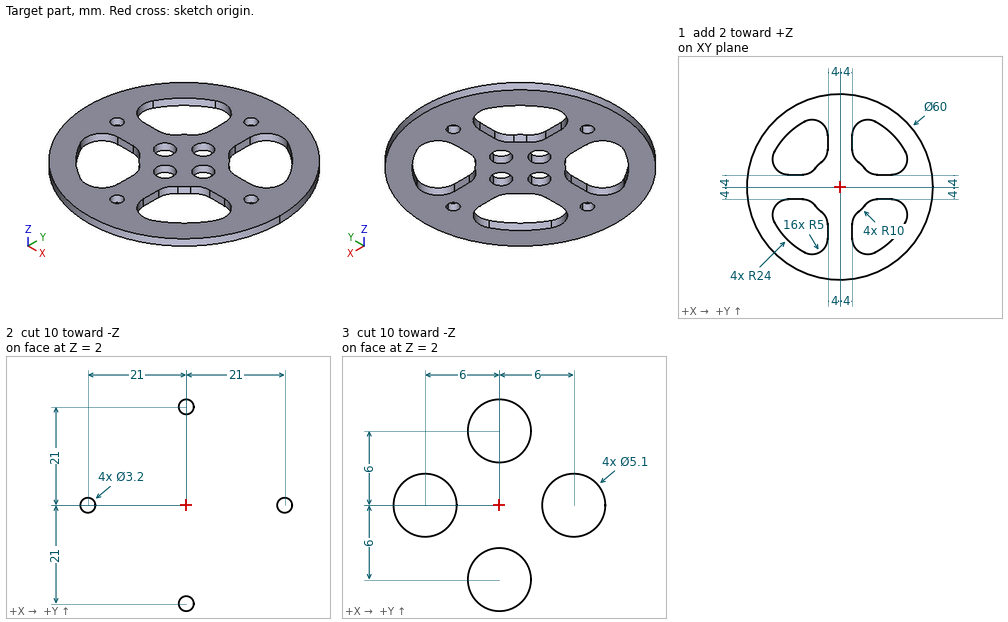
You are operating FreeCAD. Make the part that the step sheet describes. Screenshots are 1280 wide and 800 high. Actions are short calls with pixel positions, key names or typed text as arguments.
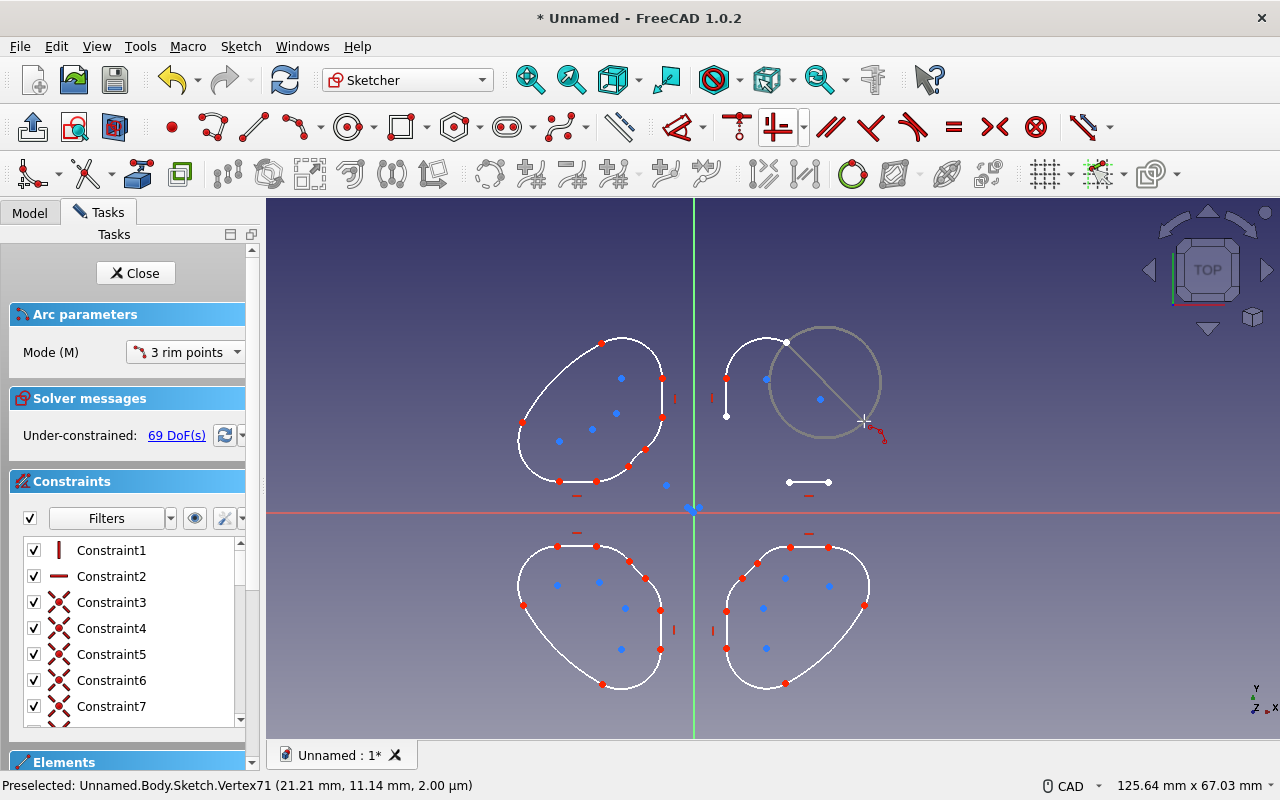
scroll(831, 376, up, 4)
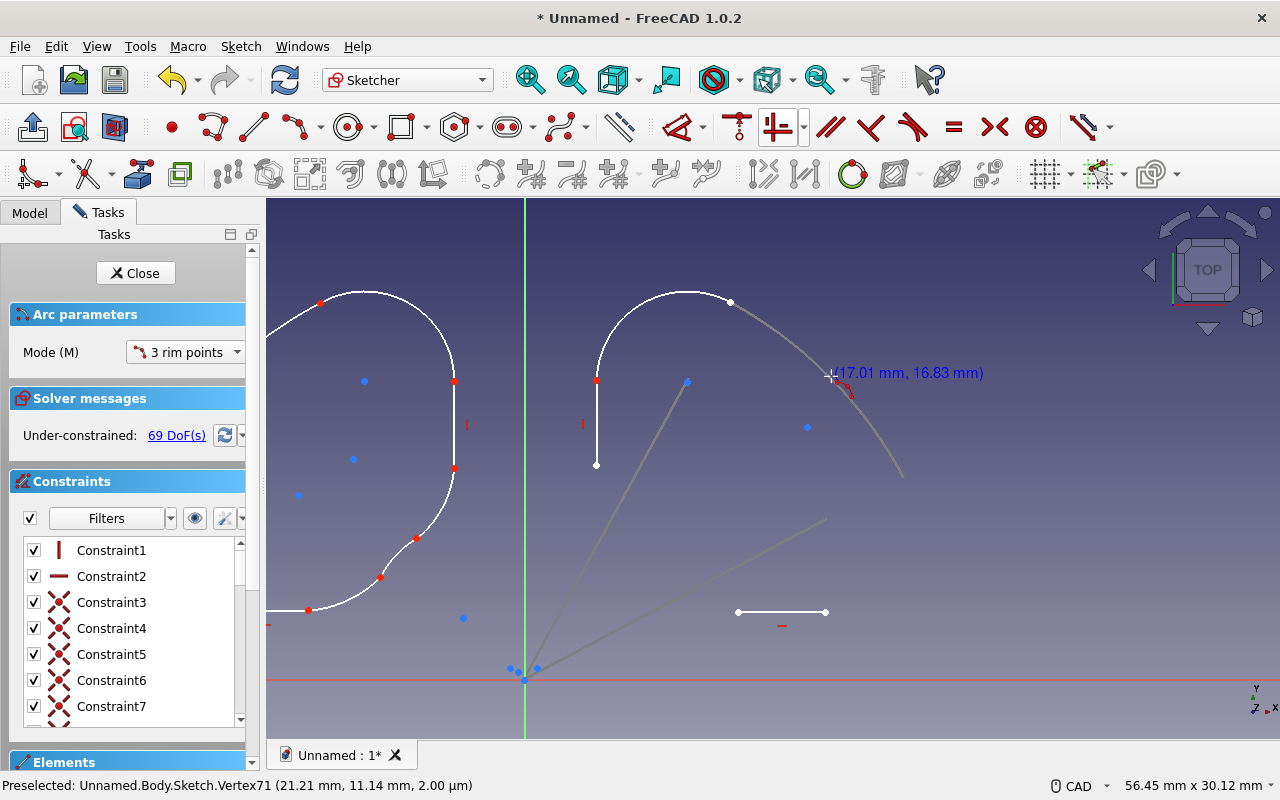
click(830, 375)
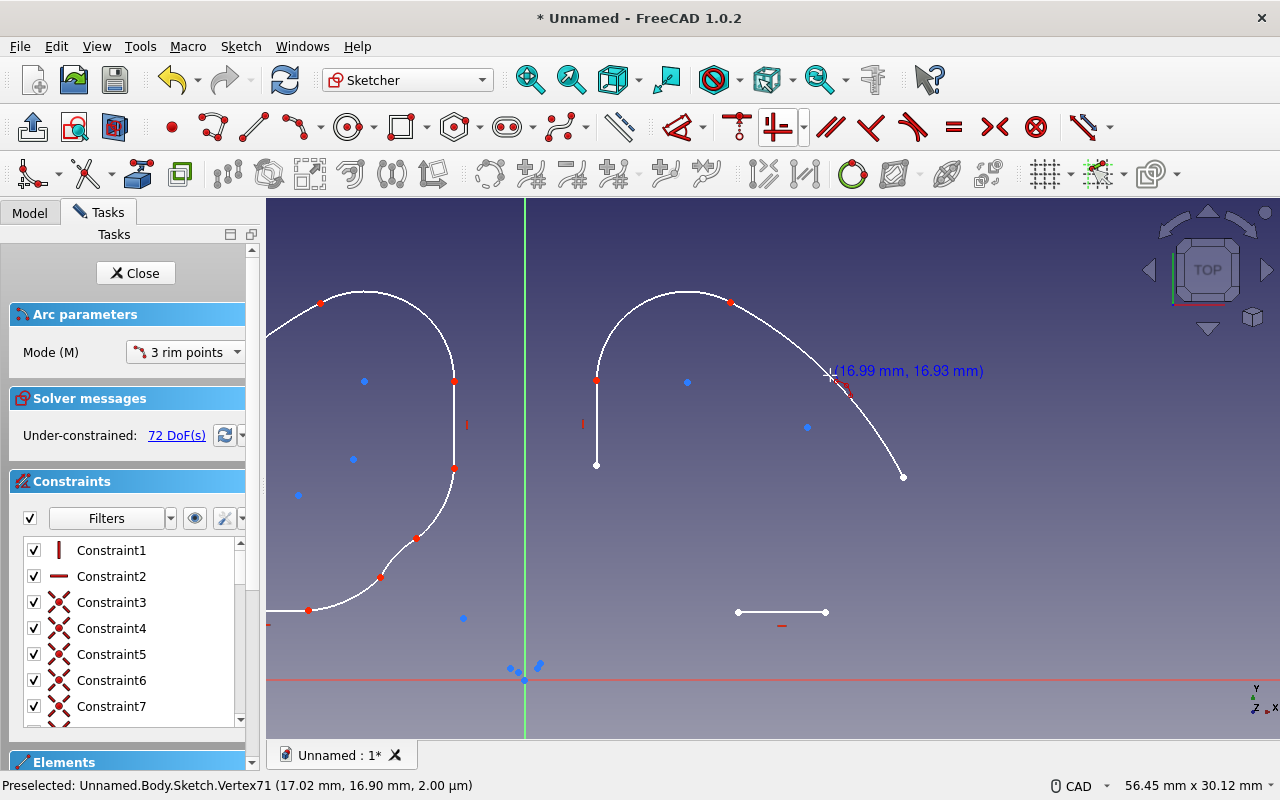
click(904, 478)
click(825, 612)
click(903, 565)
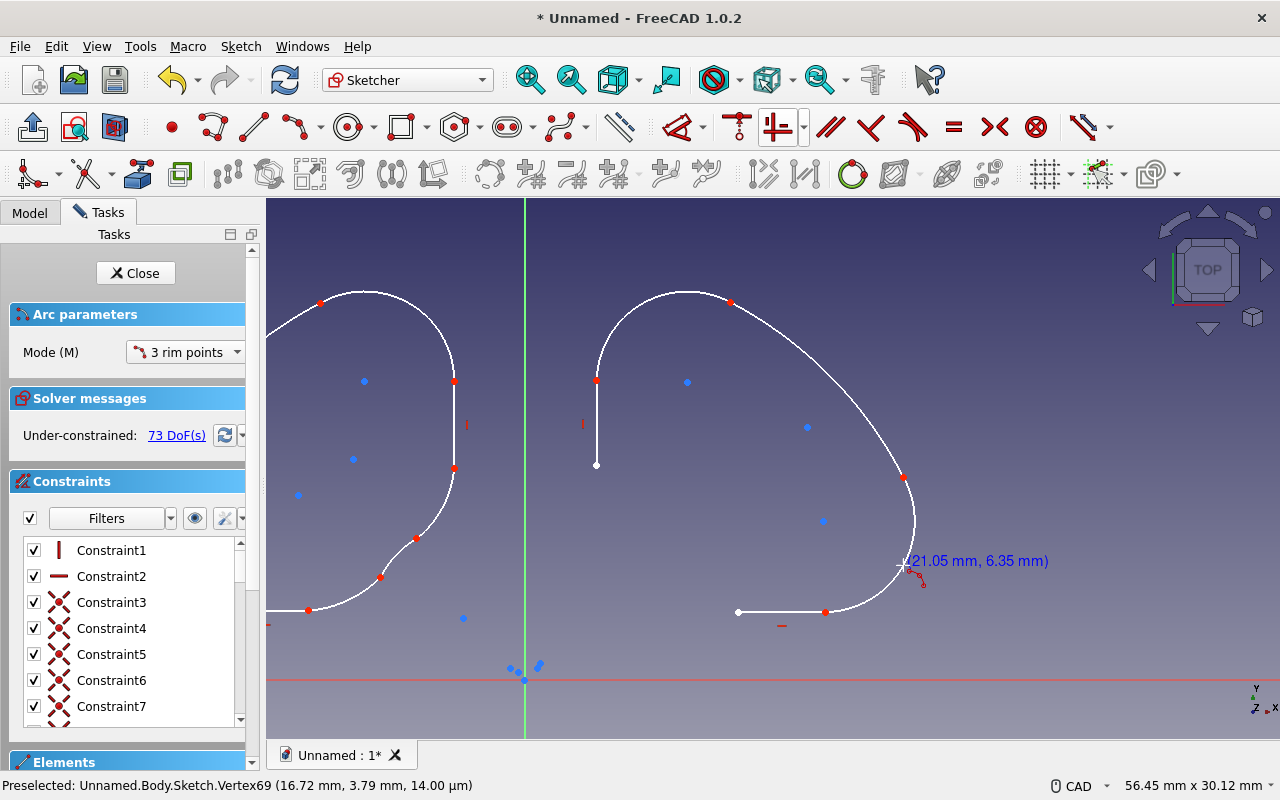
click(739, 612)
click(669, 572)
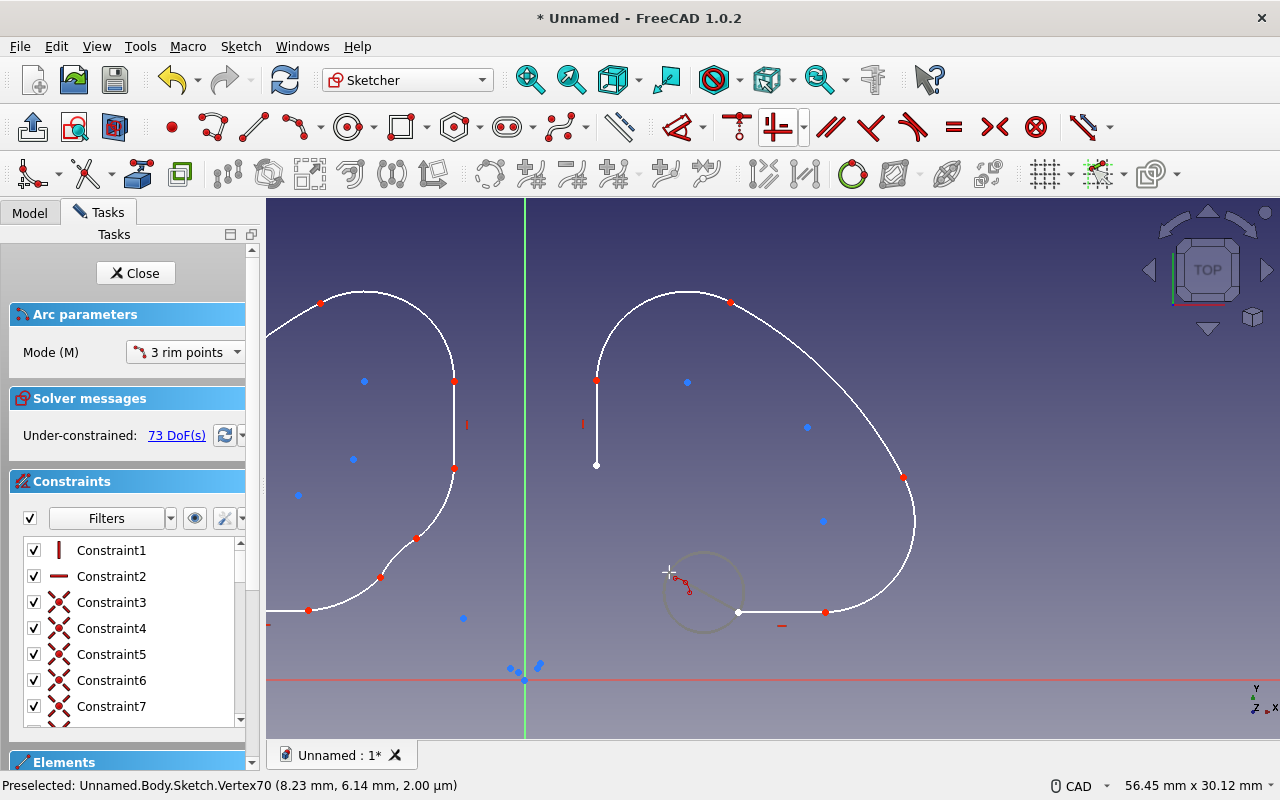
scroll(700, 599, up, 3)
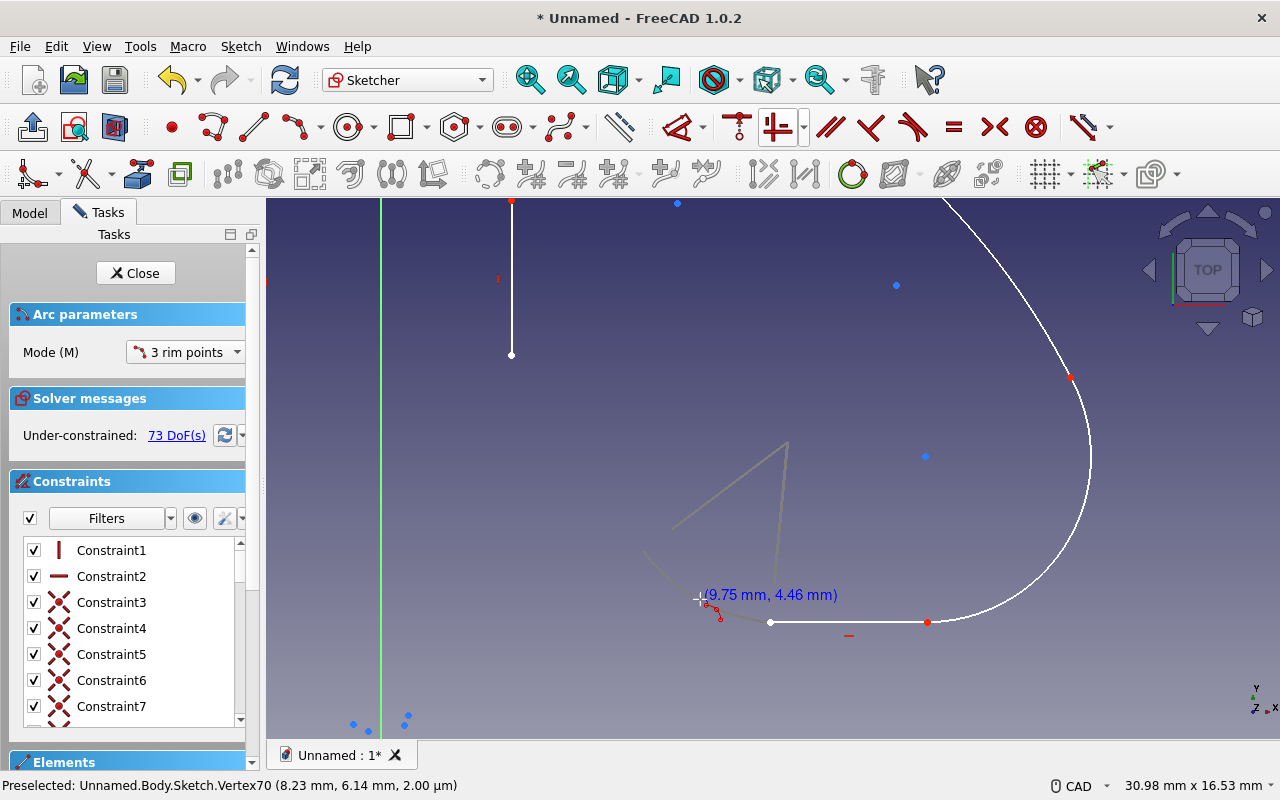
click(700, 598)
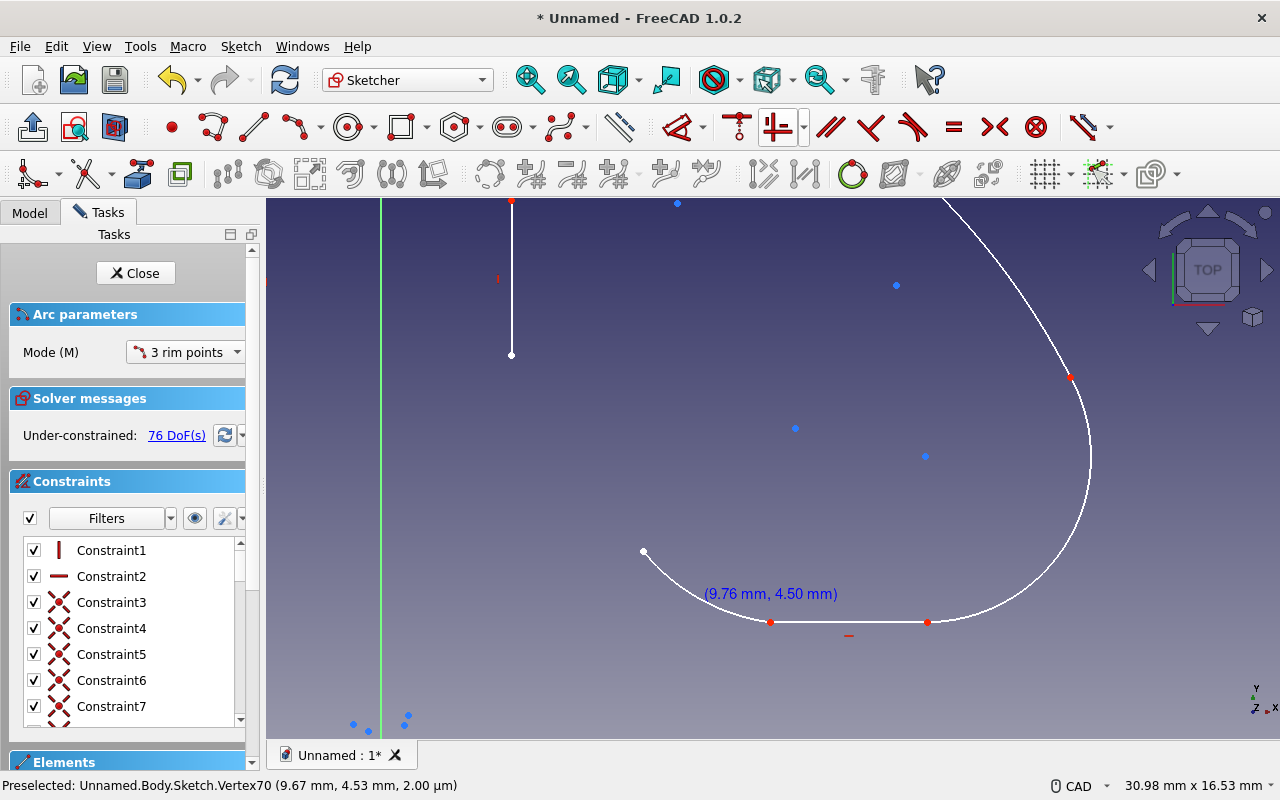
scroll(769, 414, down, 9)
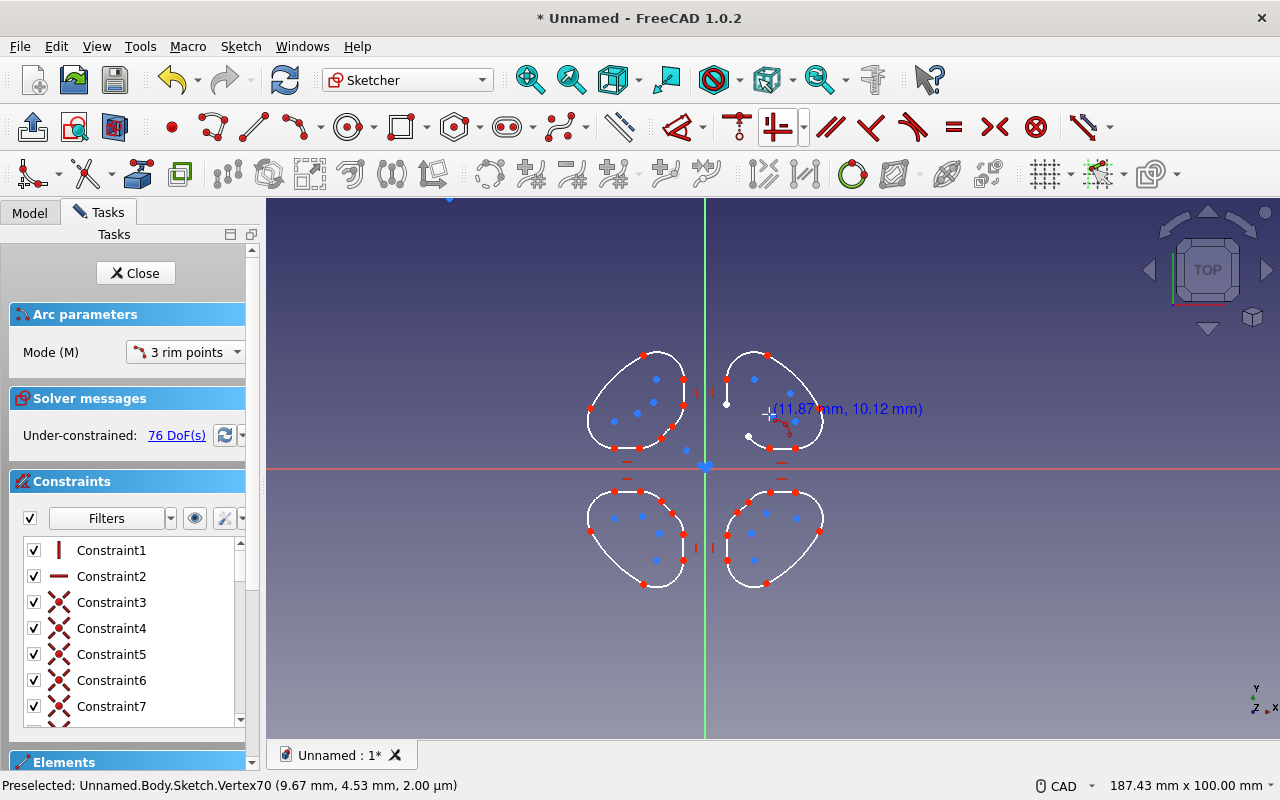
click(749, 437)
click(738, 426)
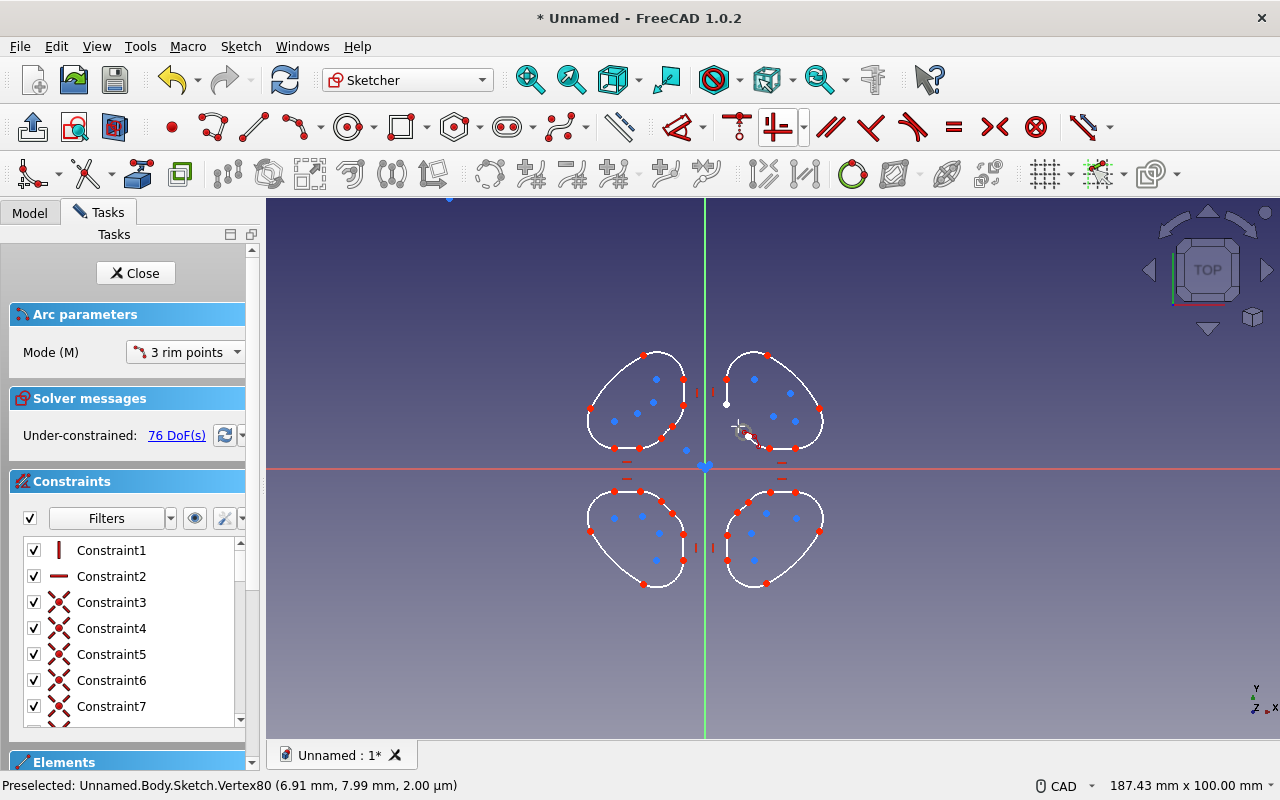
scroll(743, 431, up, 17)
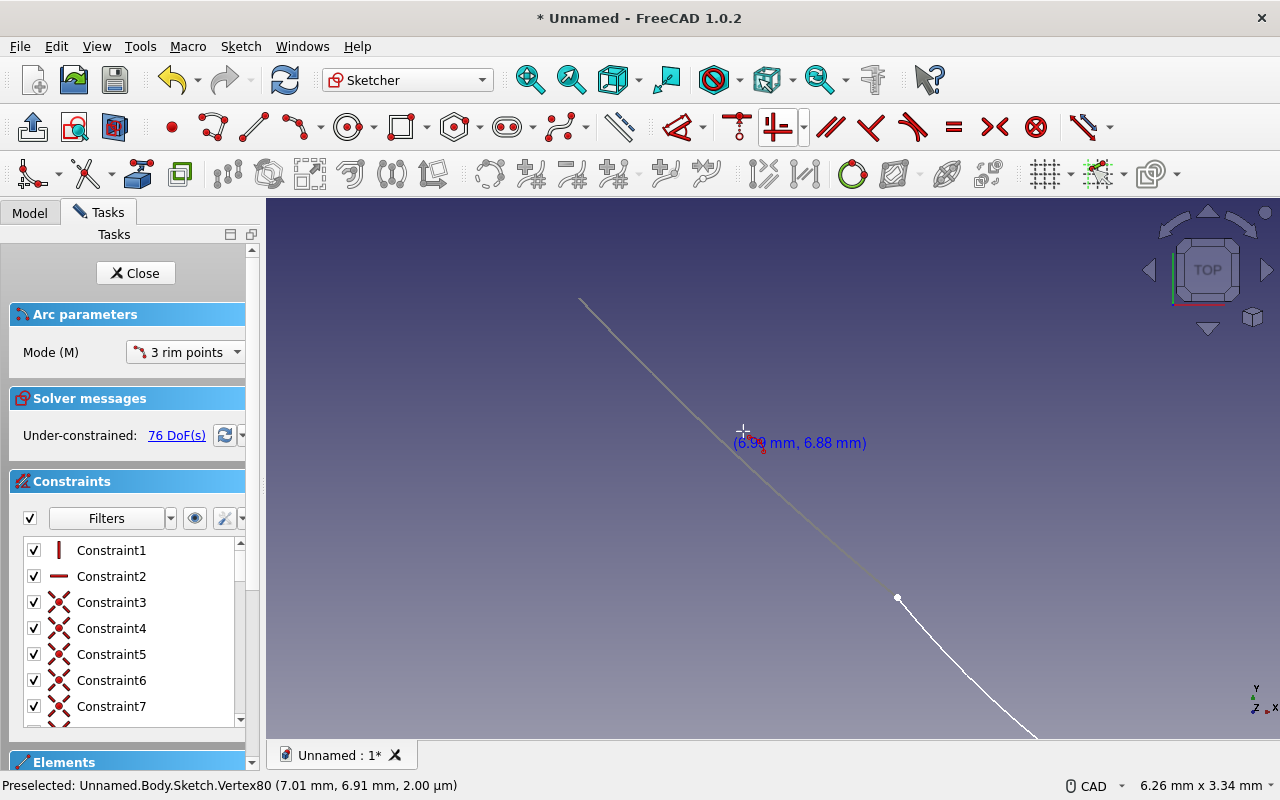
click(743, 418)